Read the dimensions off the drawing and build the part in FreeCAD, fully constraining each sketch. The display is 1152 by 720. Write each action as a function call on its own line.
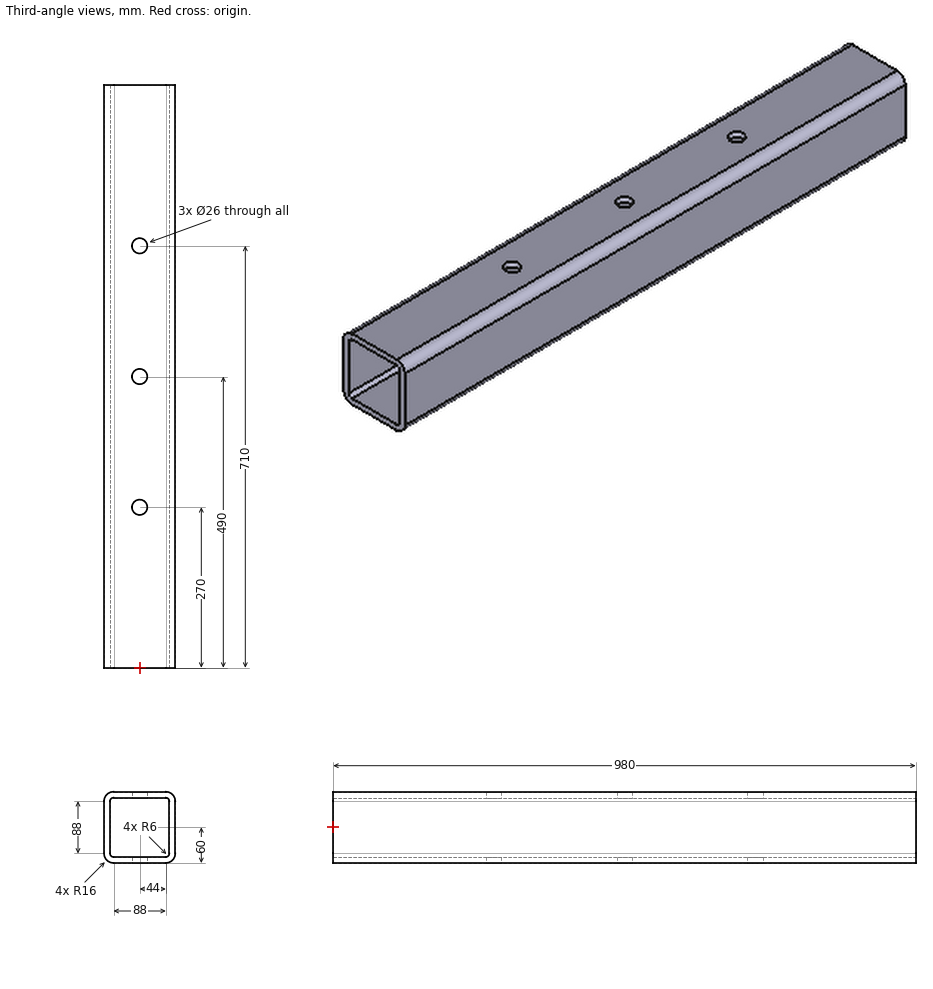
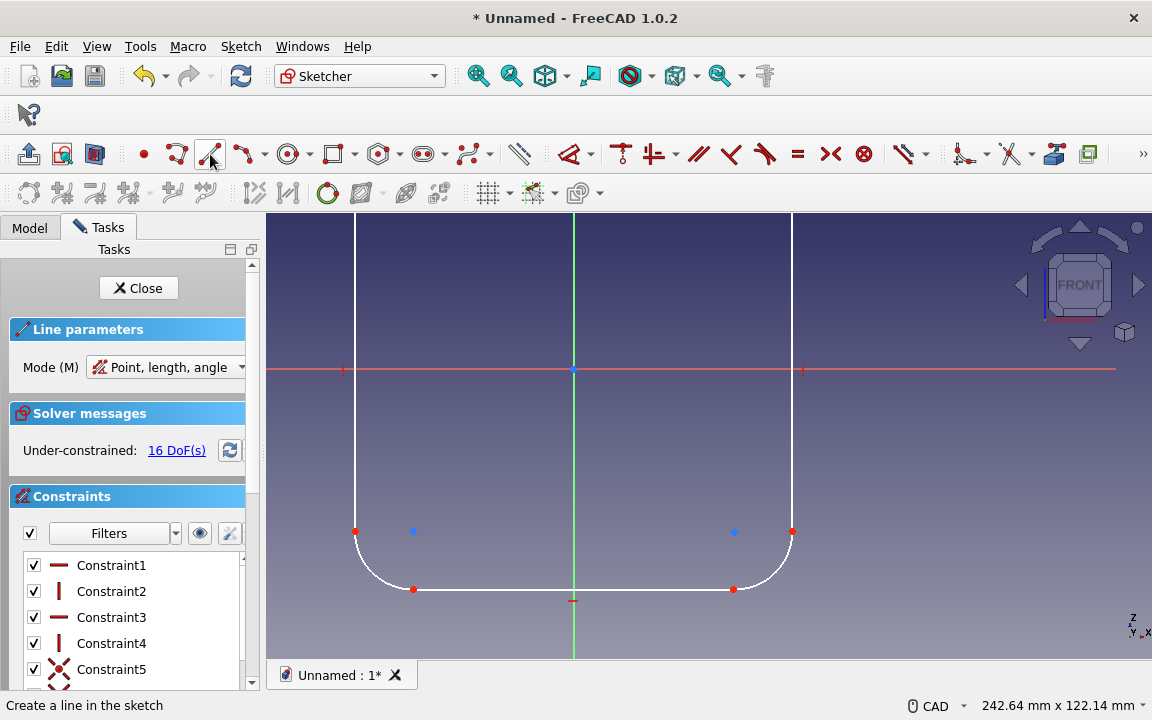
click(413, 552)
click(734, 552)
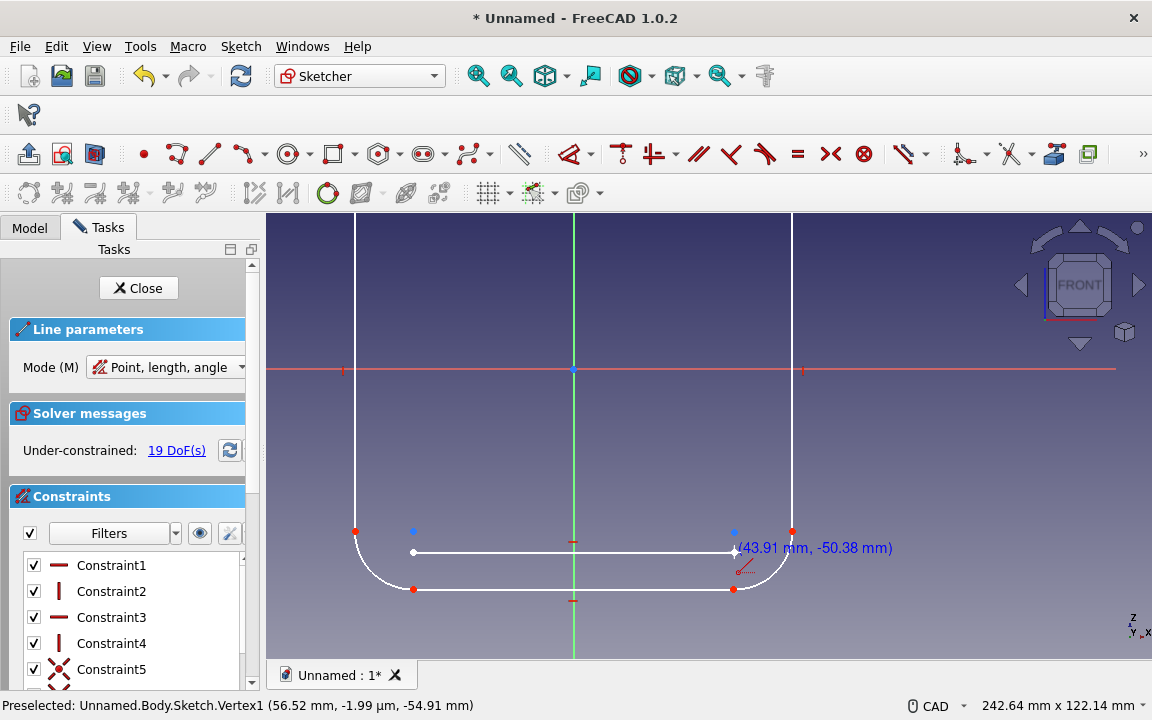
click(756, 530)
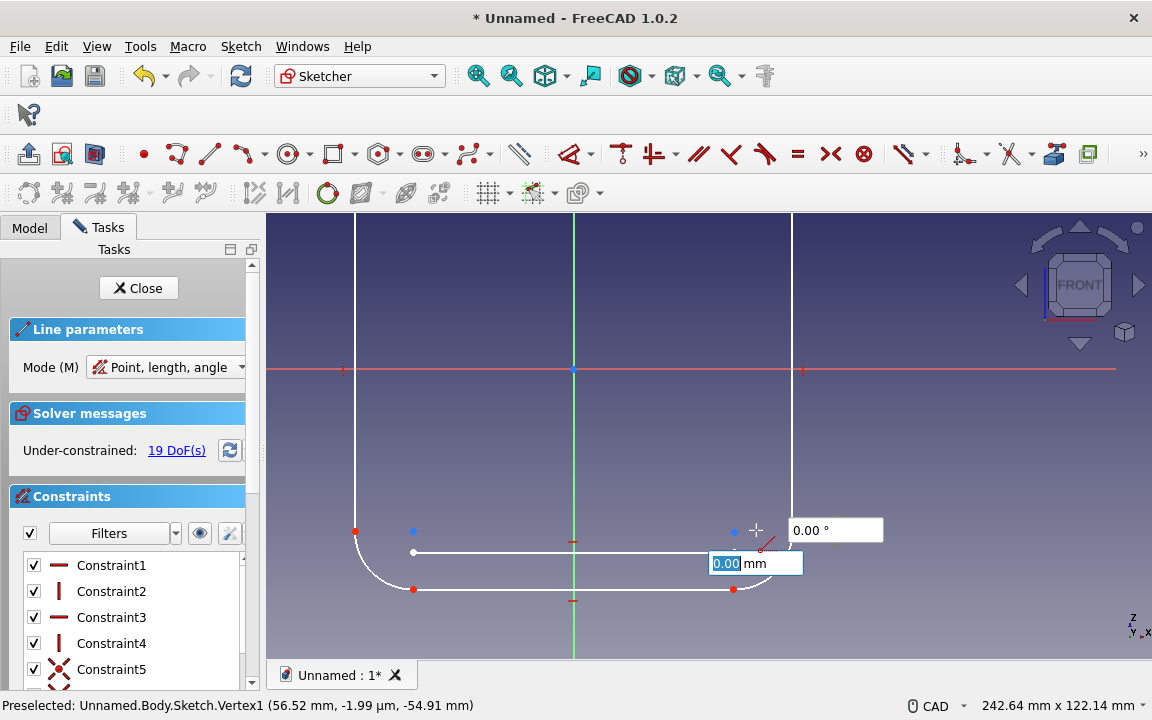
scroll(776, 572, down, 2)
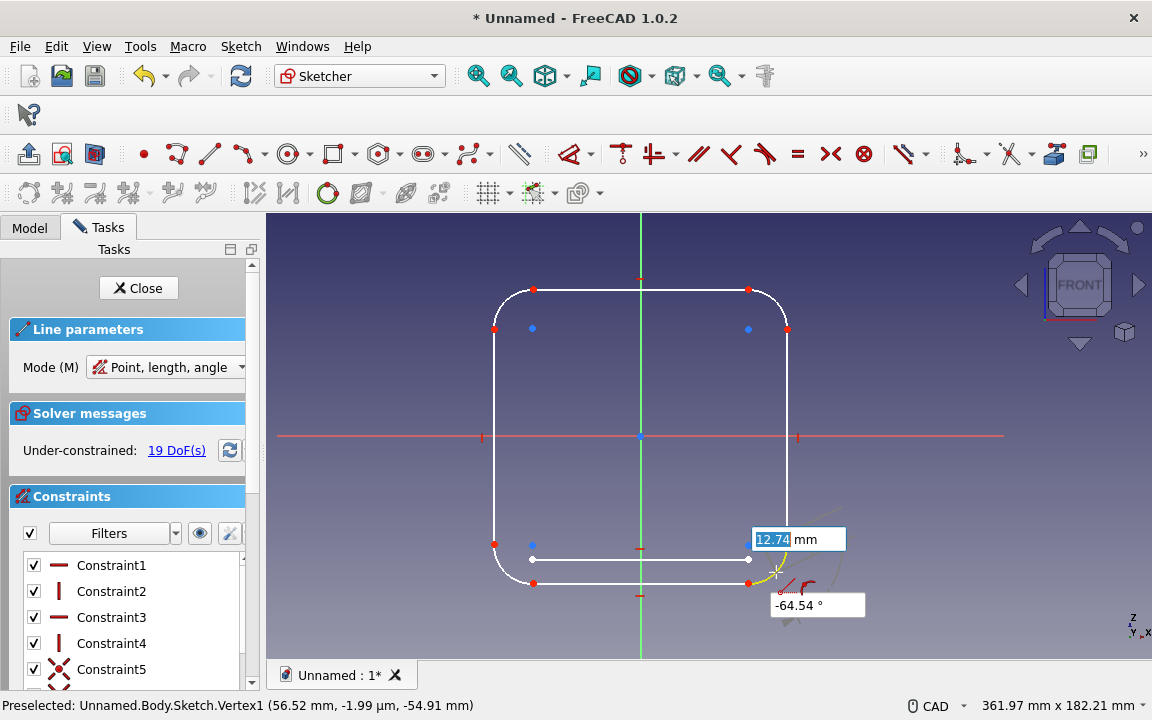
click(763, 329)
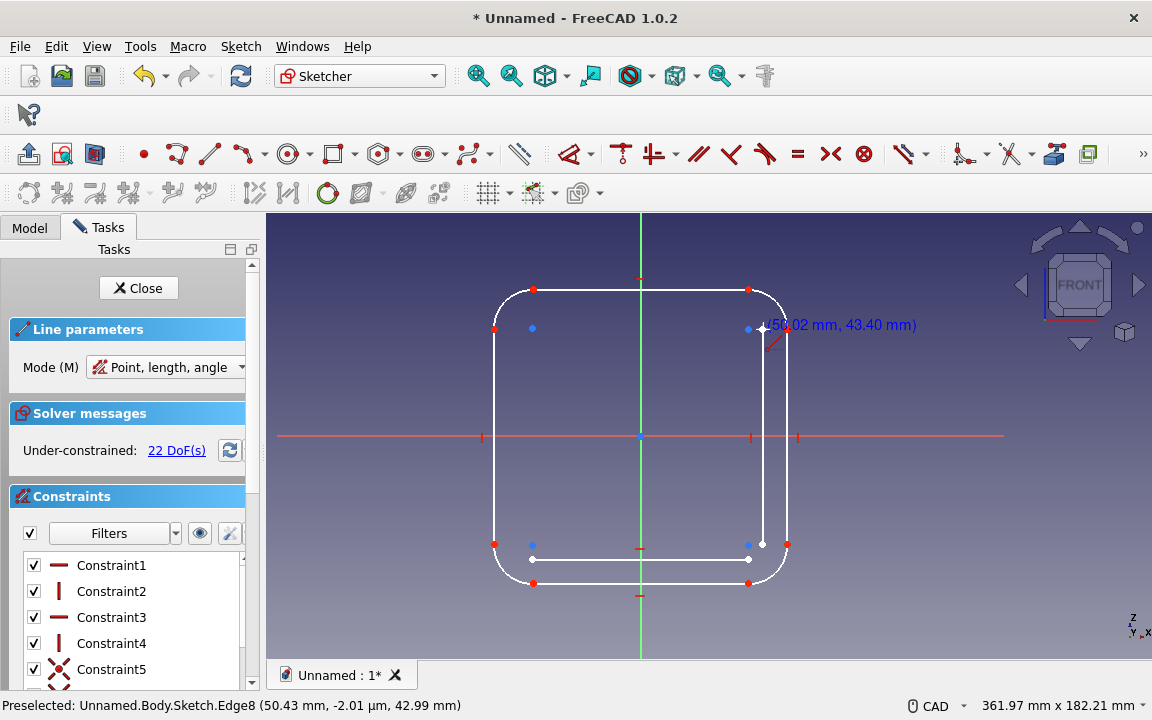
click(748, 314)
click(533, 314)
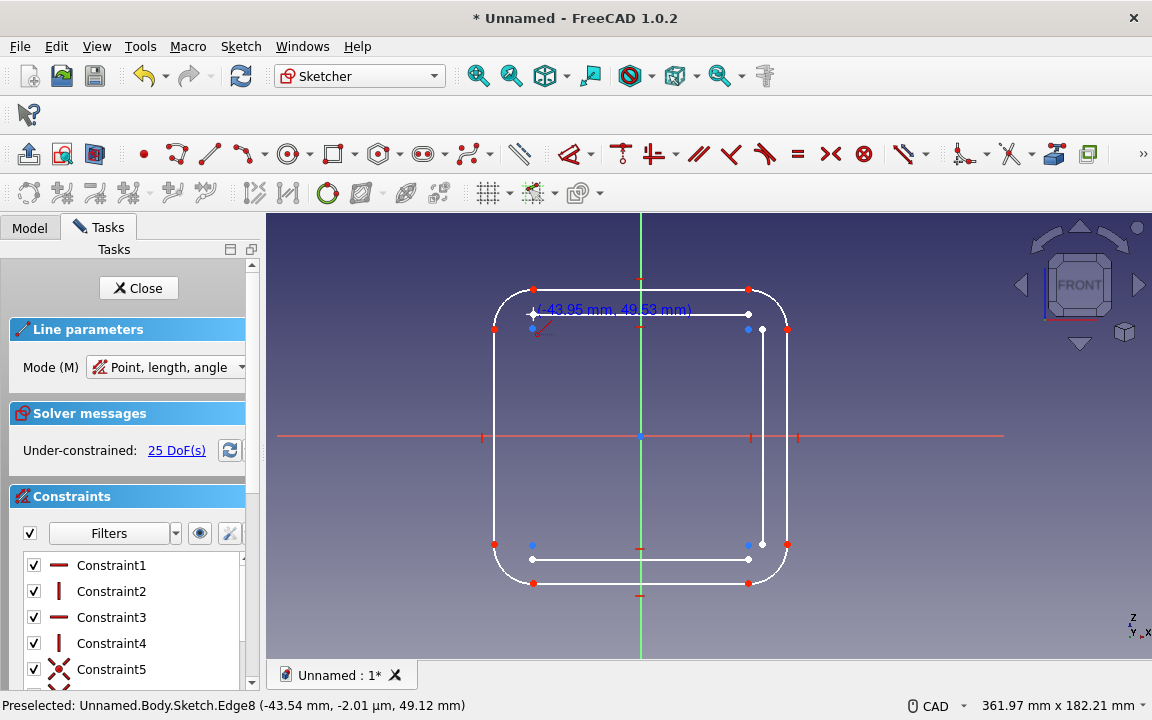
click(518, 329)
click(518, 544)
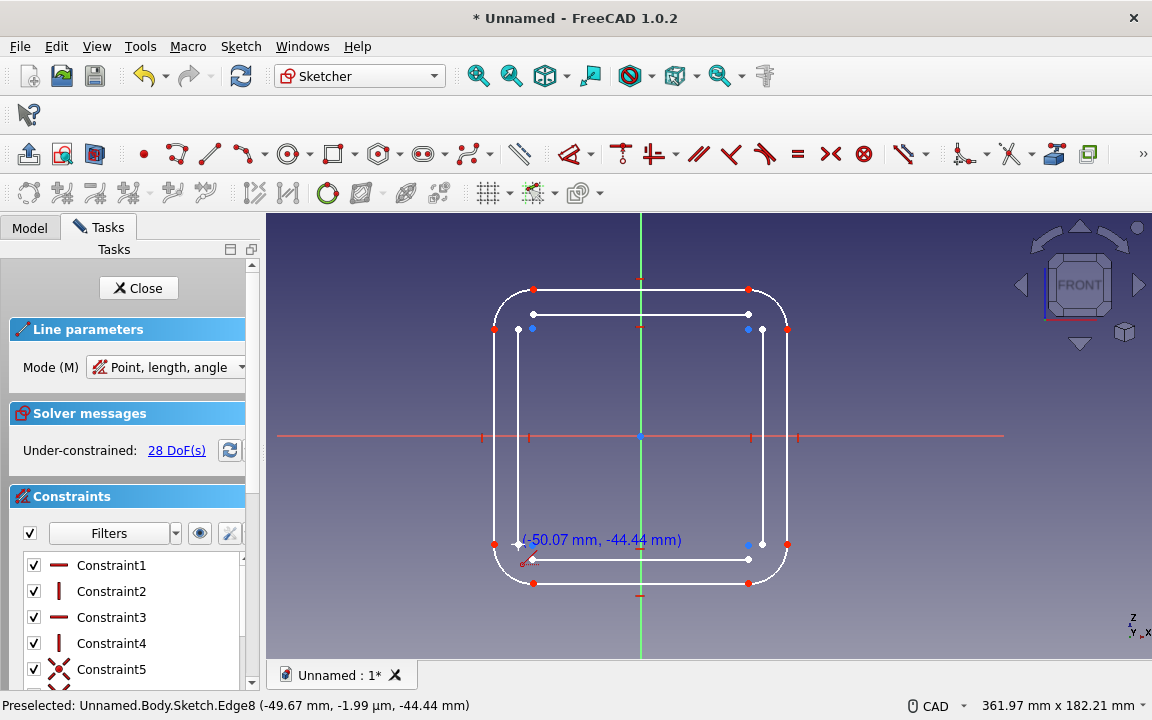
click(242, 154)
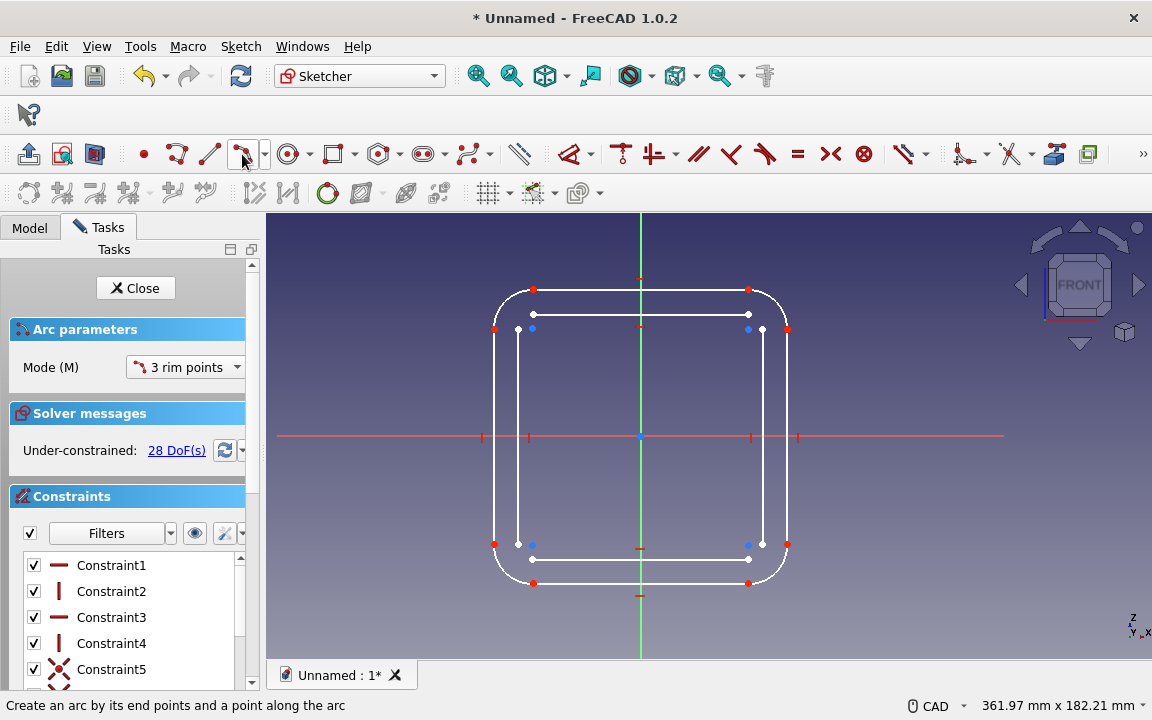
click(748, 560)
click(763, 545)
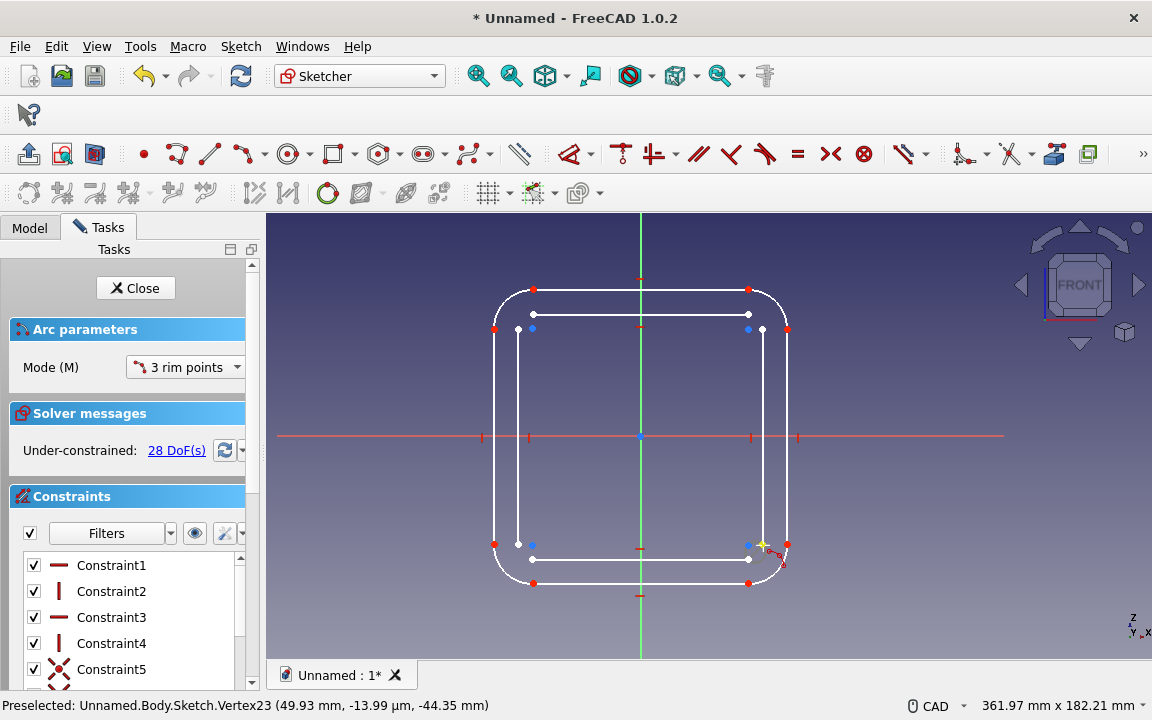
scroll(759, 554, up, 7)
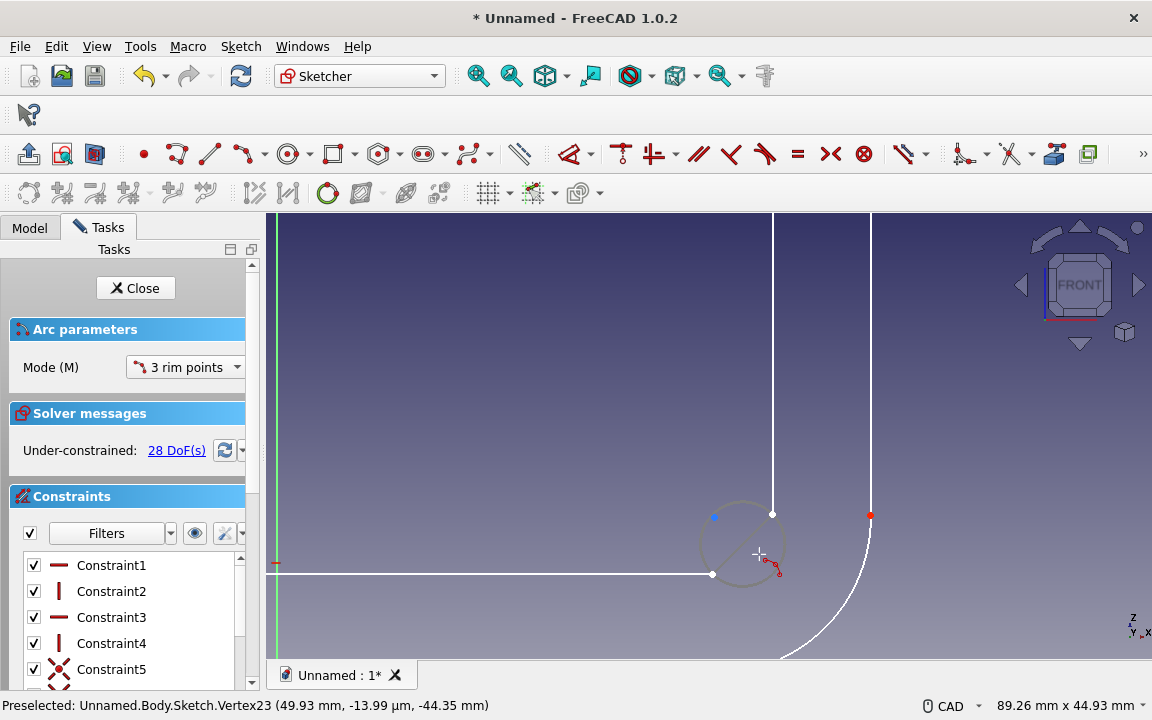
click(756, 553)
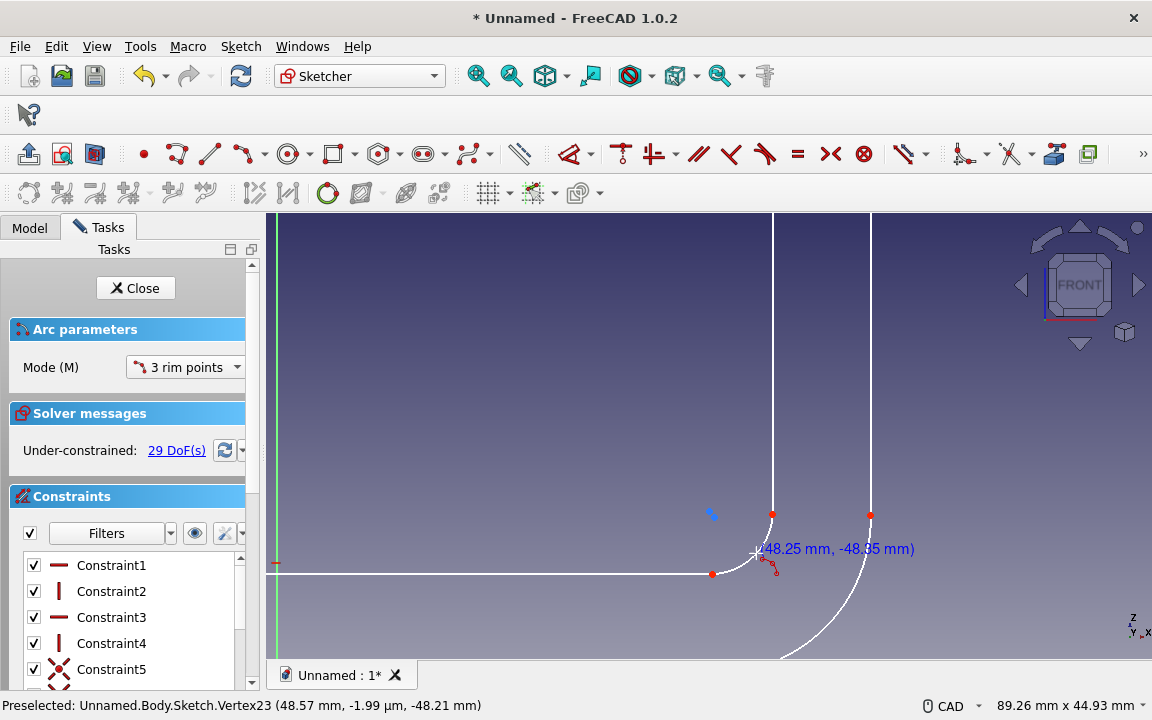
scroll(759, 554, down, 7)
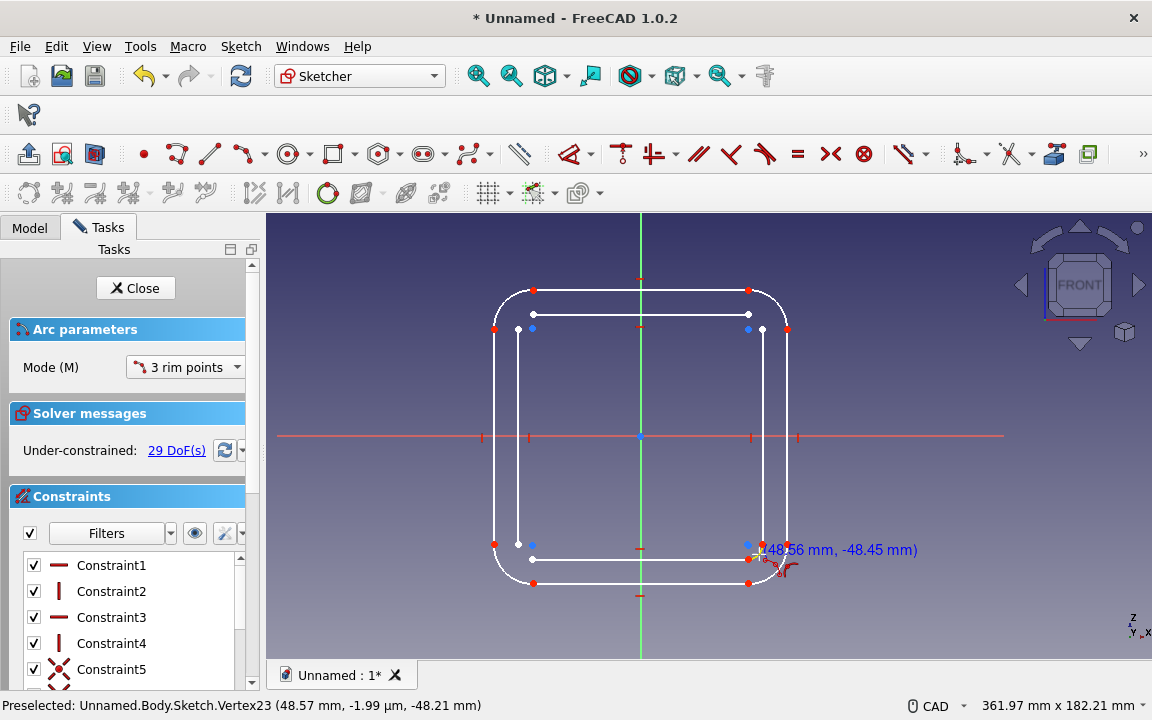
click(763, 330)
click(748, 315)